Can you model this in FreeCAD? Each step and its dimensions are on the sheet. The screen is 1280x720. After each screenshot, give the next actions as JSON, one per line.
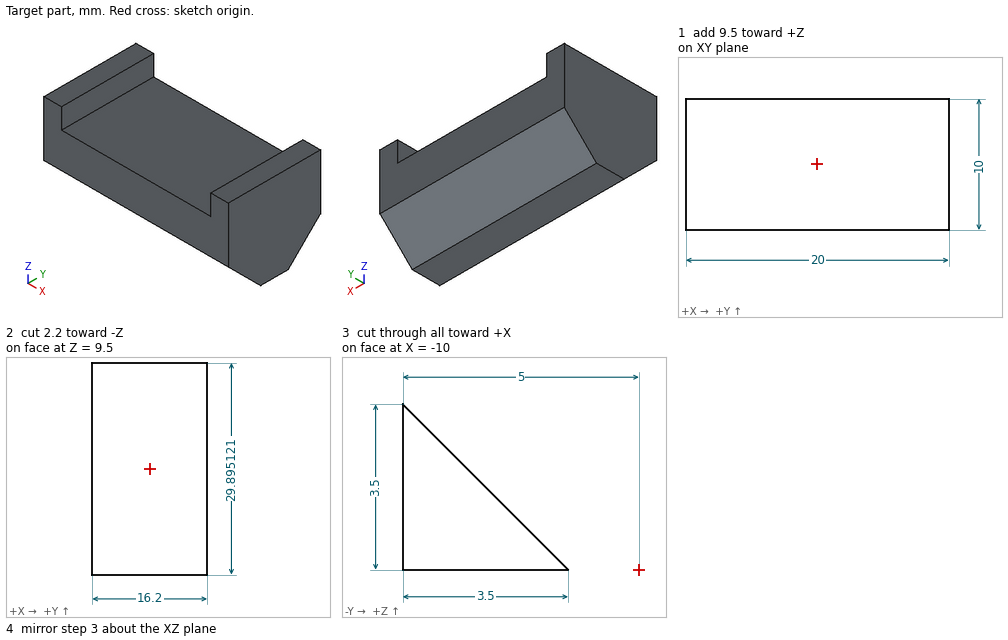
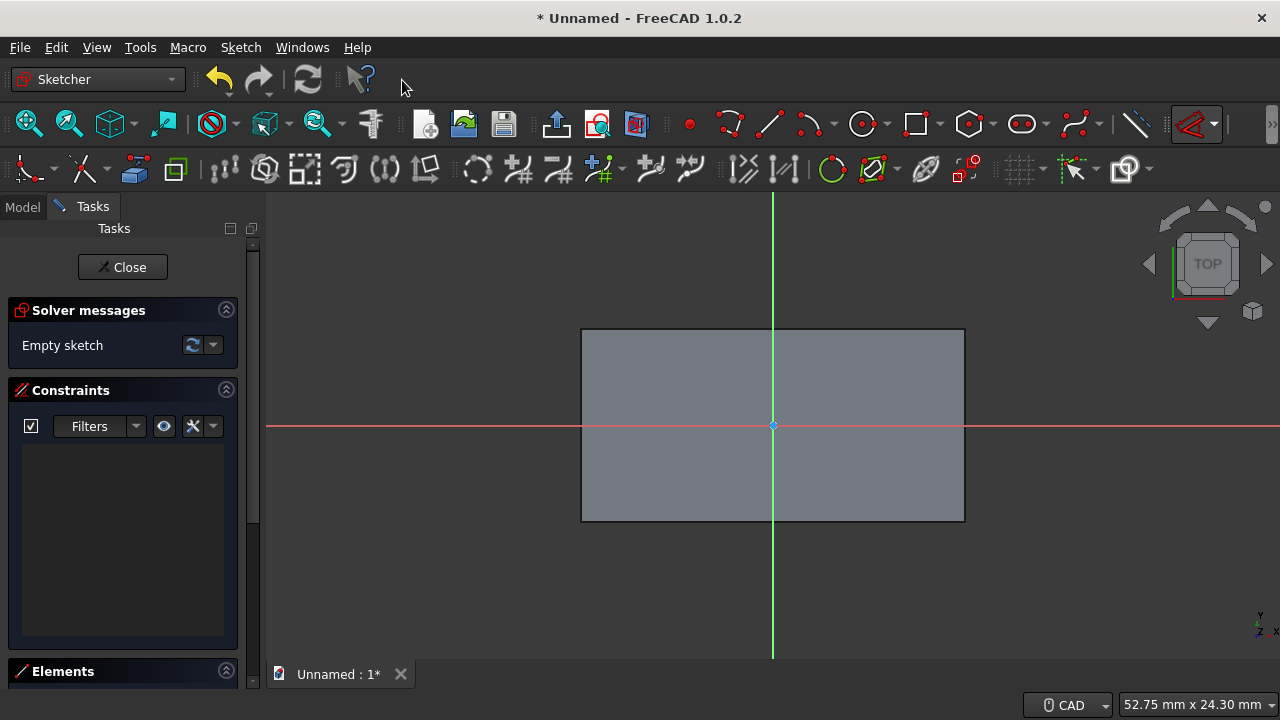
{"action": "scroll", "coordinate": [621, 426], "scroll_direction": "down", "scroll_amount": 3}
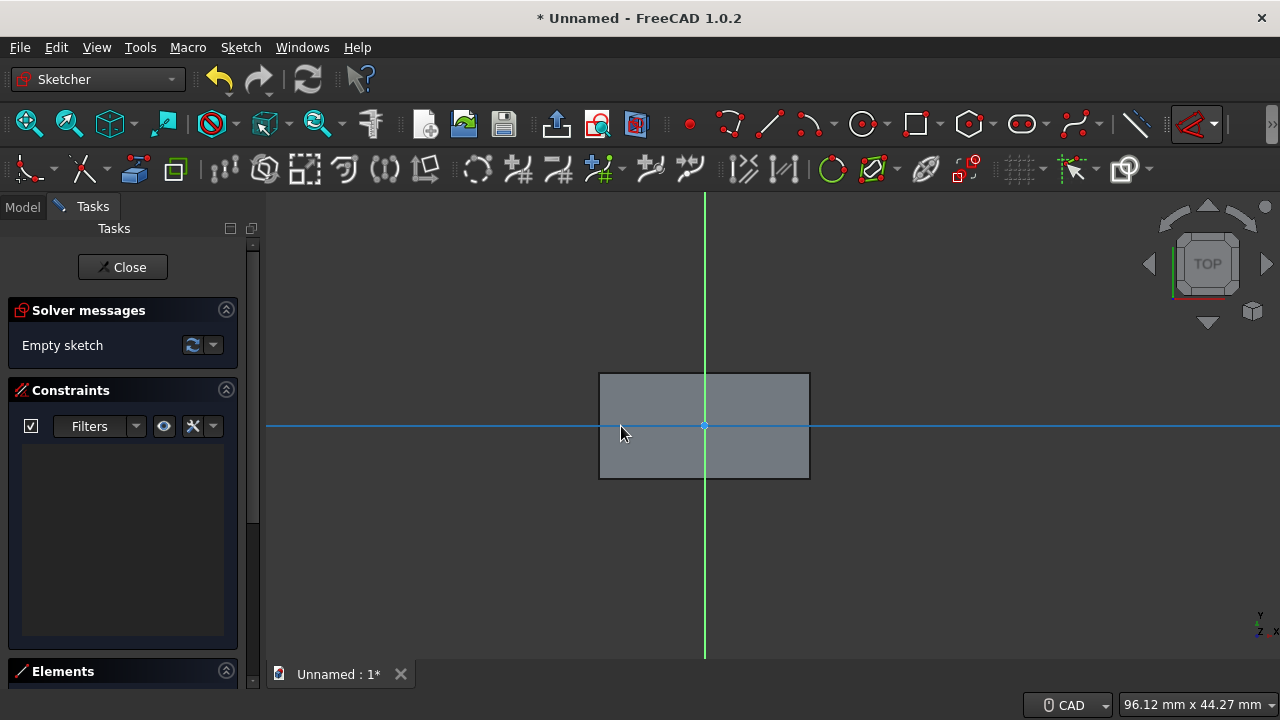
{"action": "key", "text": "g v"}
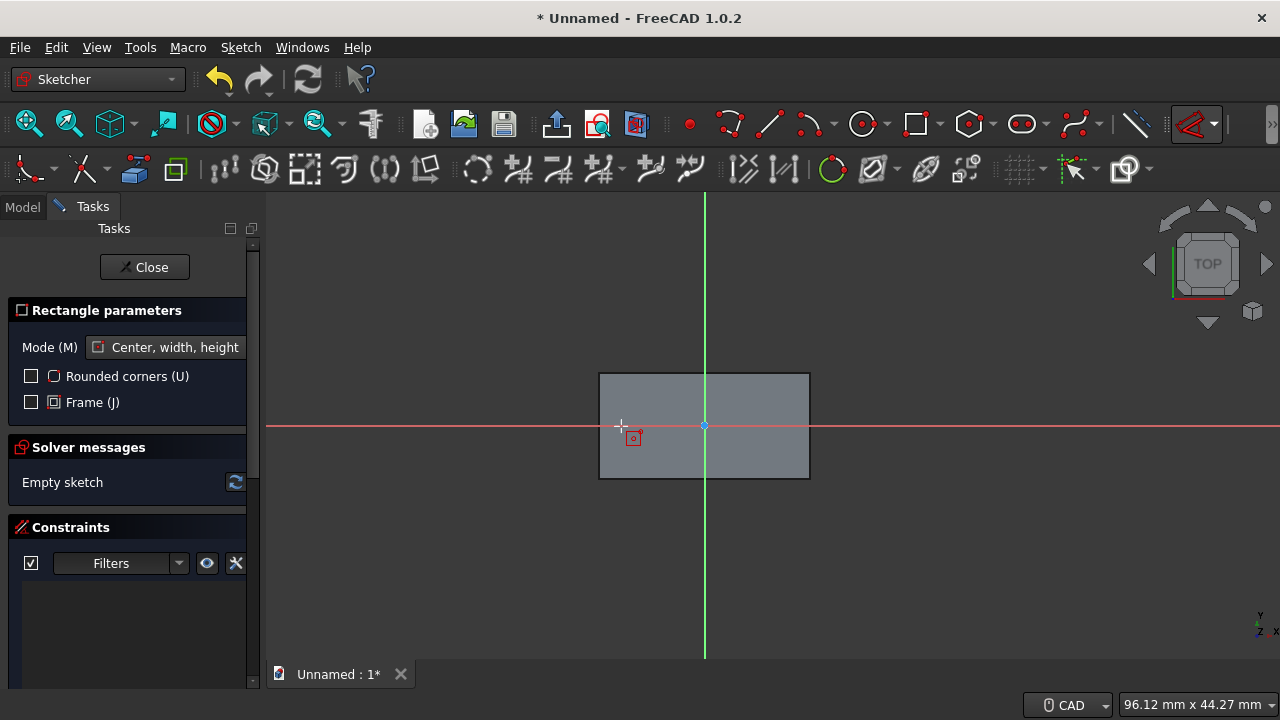
{"action": "left_click", "coordinate": [705, 426]}
{"action": "left_click", "coordinate": [790, 268]}
{"action": "key", "text": "Escape"}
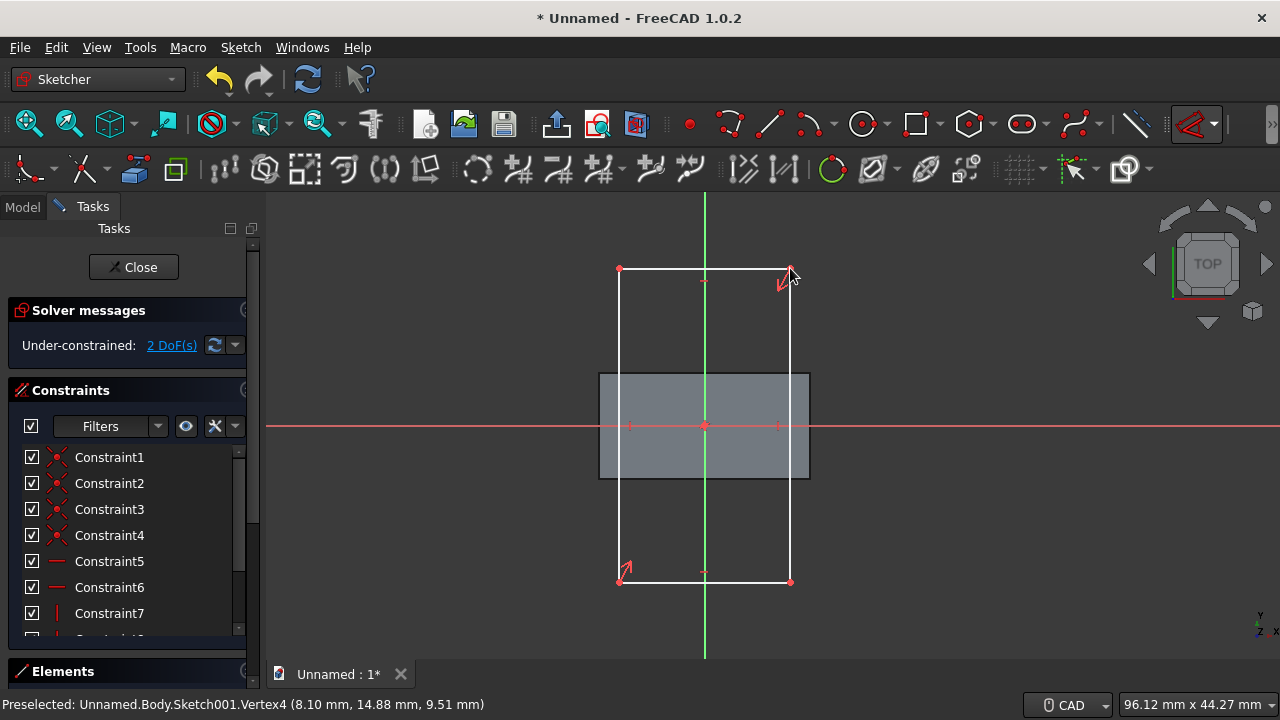
{"action": "left_click", "coordinate": [670, 583]}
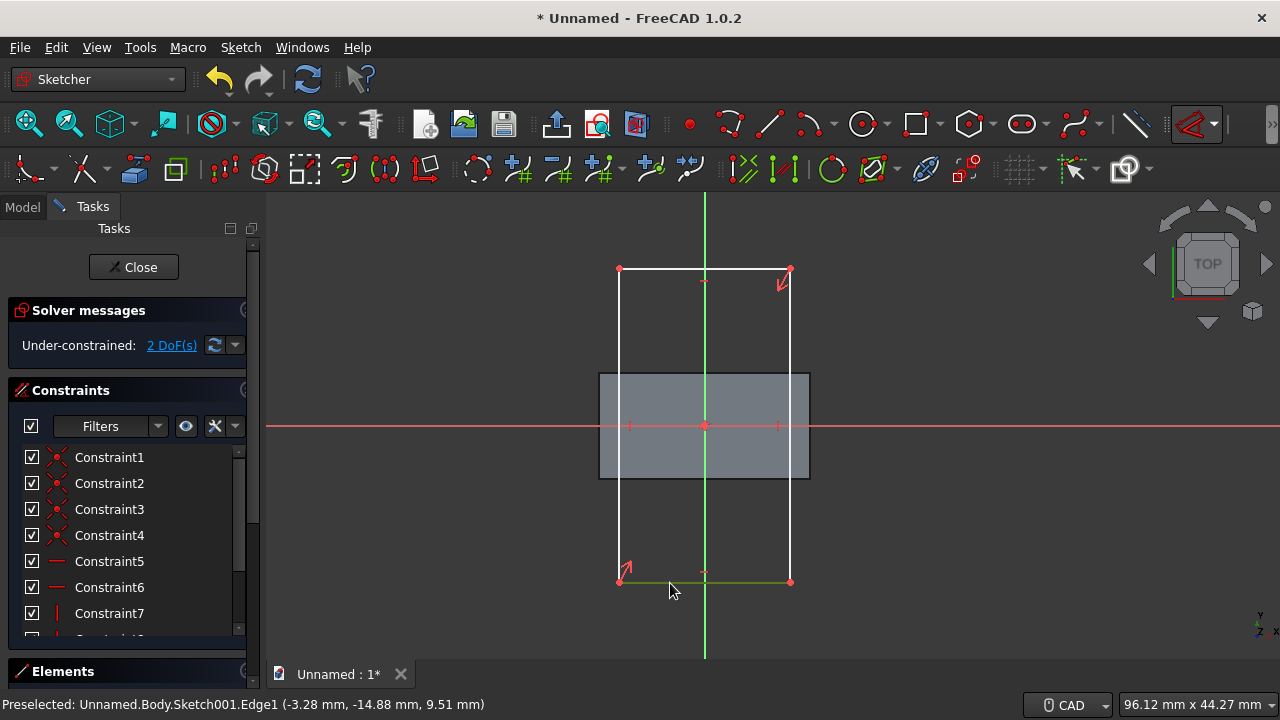
{"action": "key", "text": "l"}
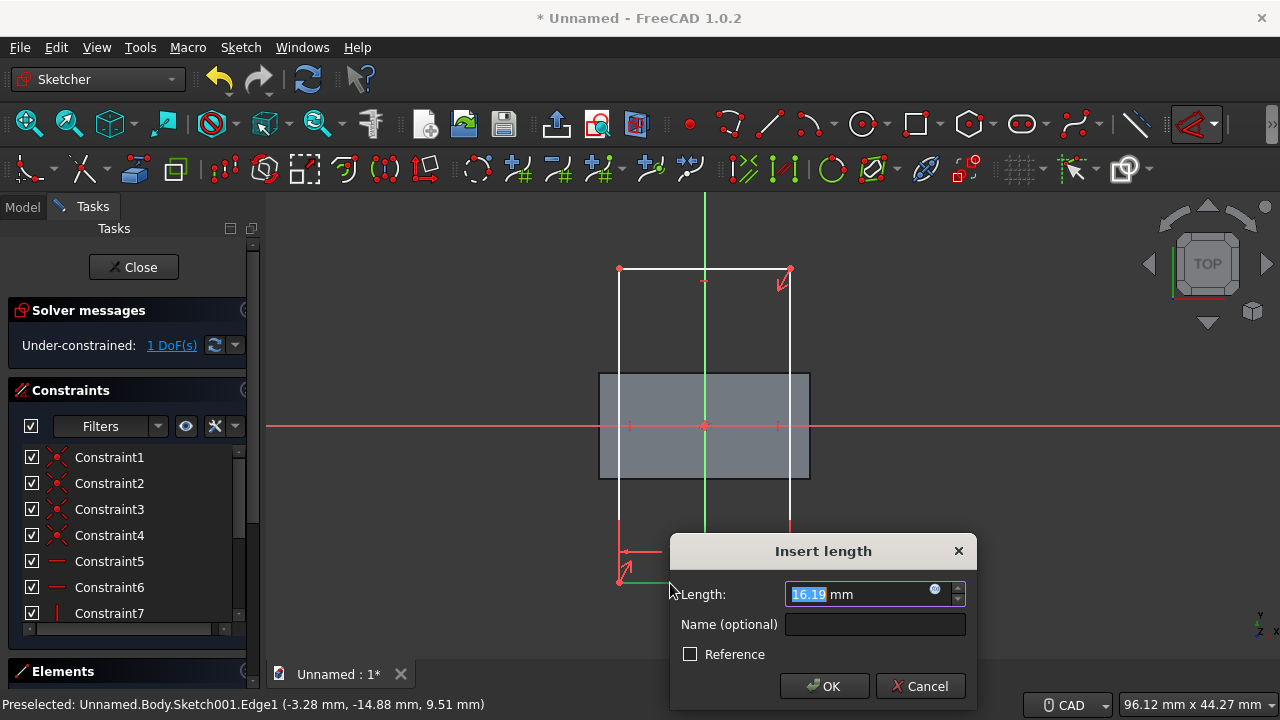
{"action": "type", "text": "16.2"}
{"action": "key", "text": "Return"}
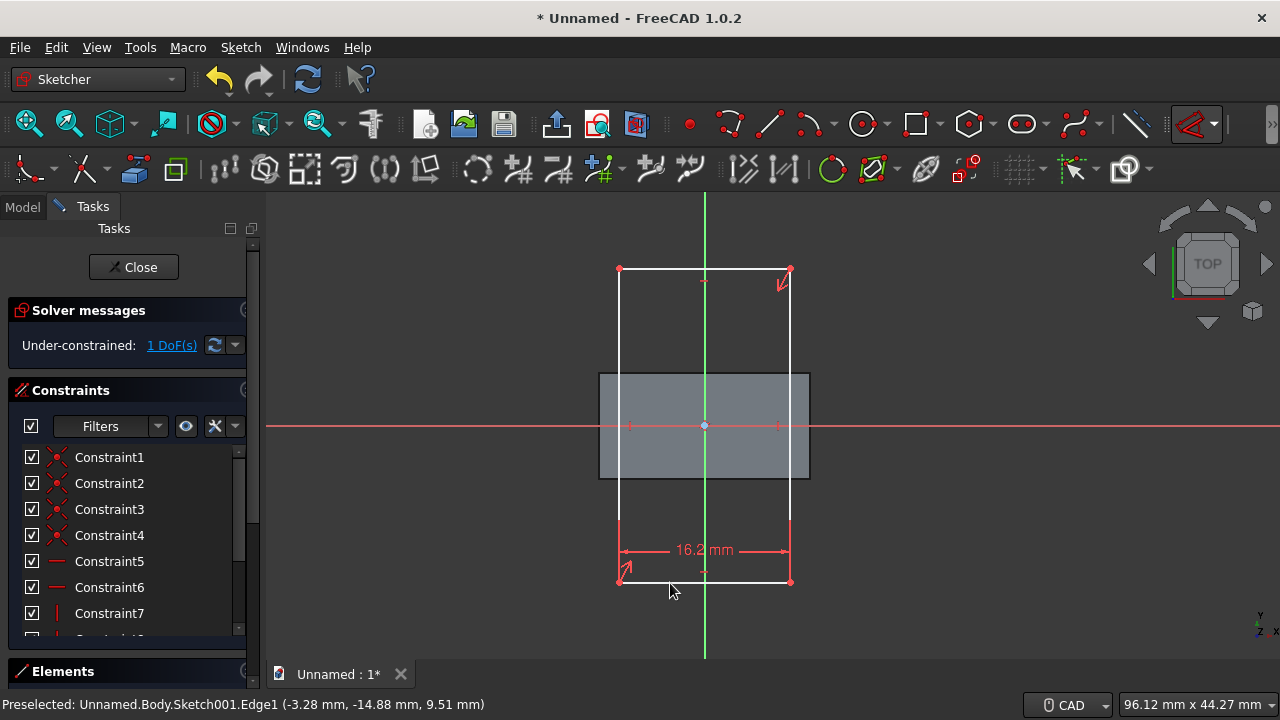
{"action": "left_click", "coordinate": [790, 489]}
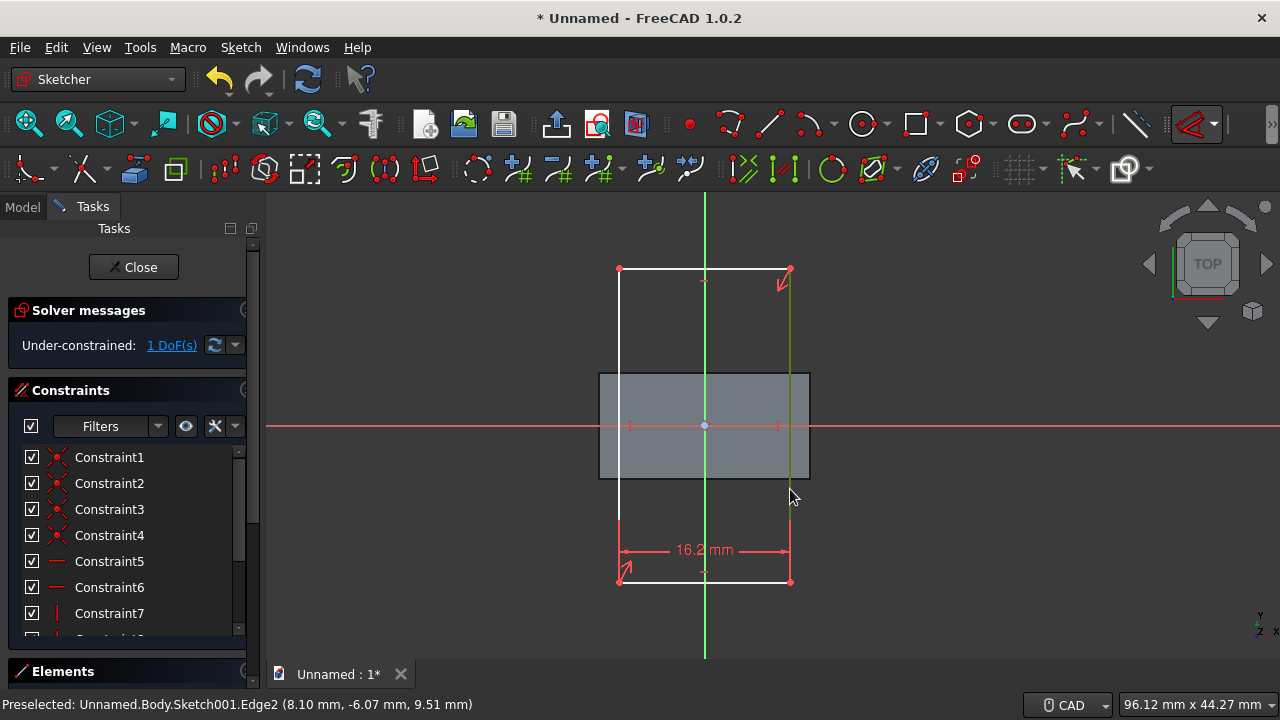
{"action": "key", "text": "i"}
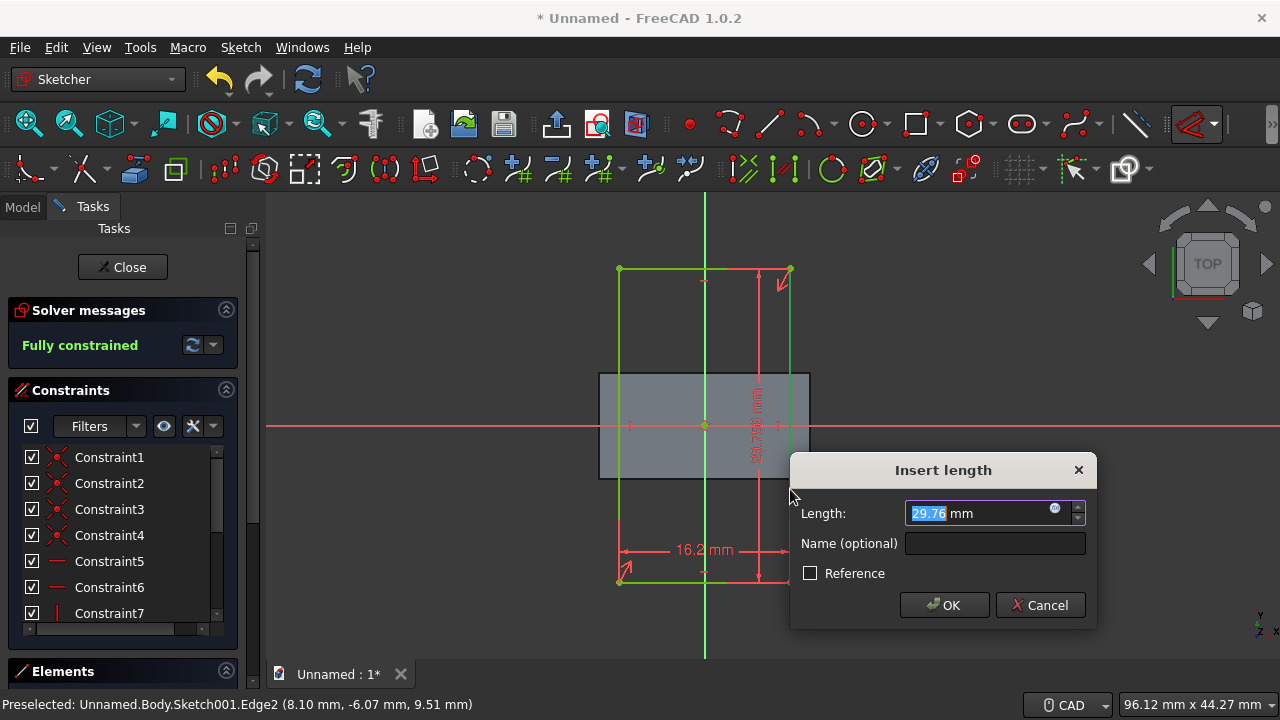
{"action": "type", "text": "29.895121"}
{"action": "key", "text": "Return"}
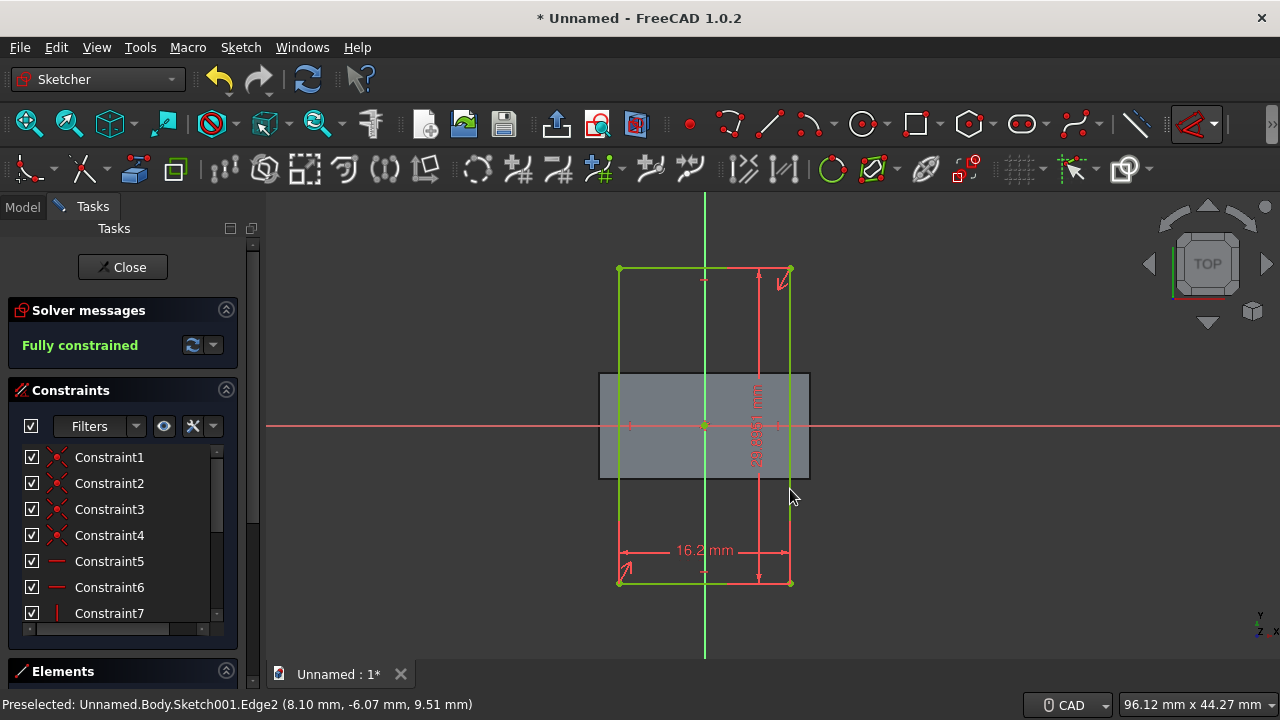
{"action": "left_click", "coordinate": [123, 267]}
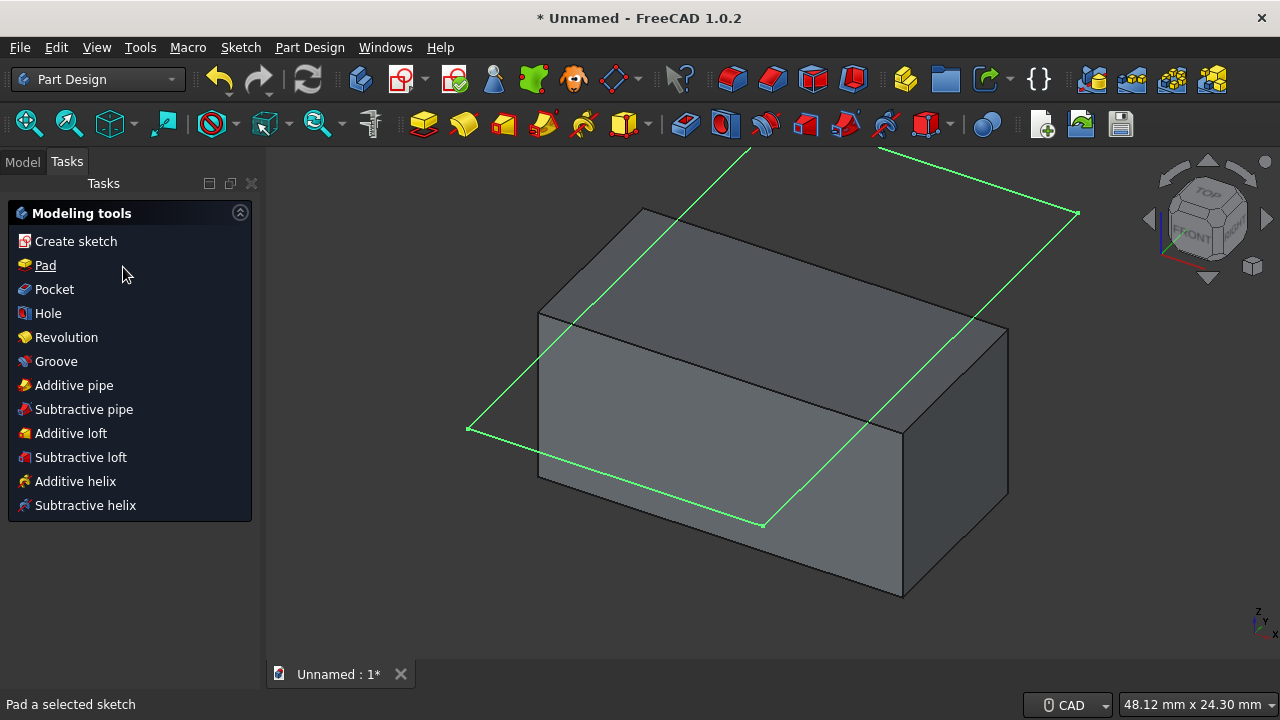
{"action": "left_click", "coordinate": [686, 124]}